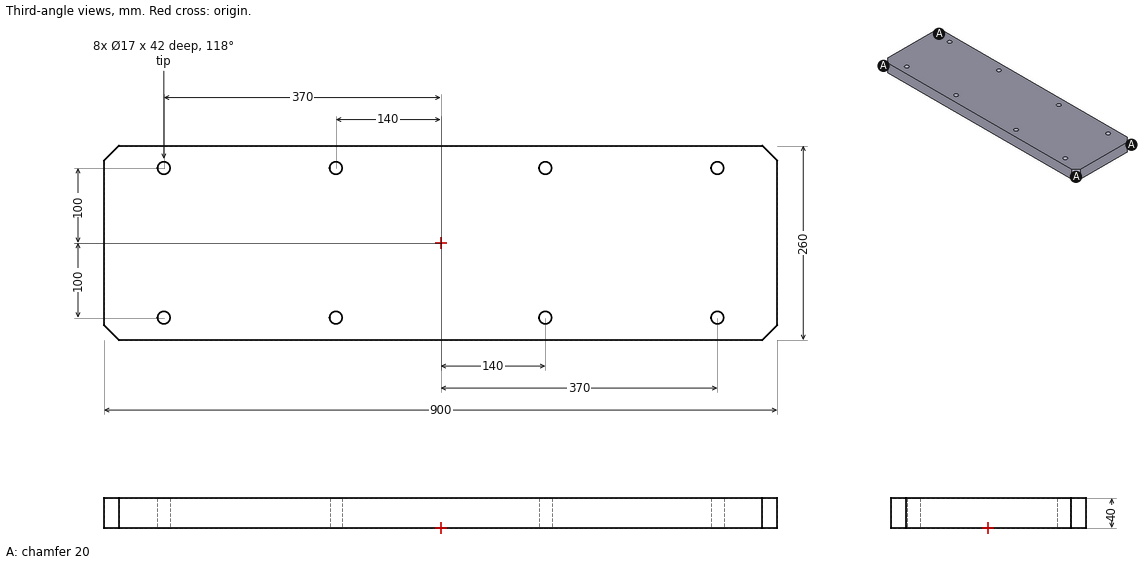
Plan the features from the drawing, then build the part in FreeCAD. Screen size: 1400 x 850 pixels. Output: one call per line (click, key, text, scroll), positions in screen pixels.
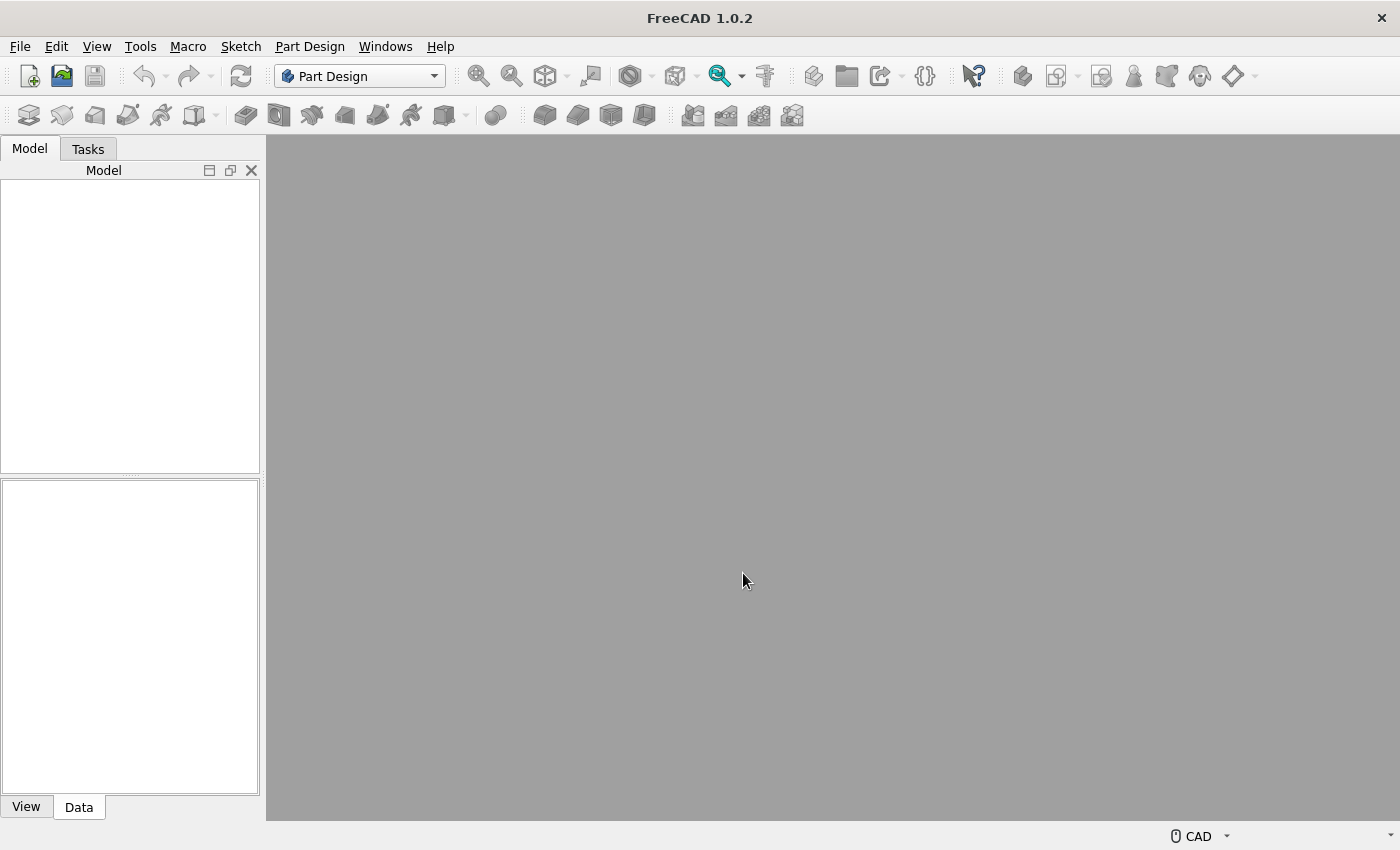
click(29, 76)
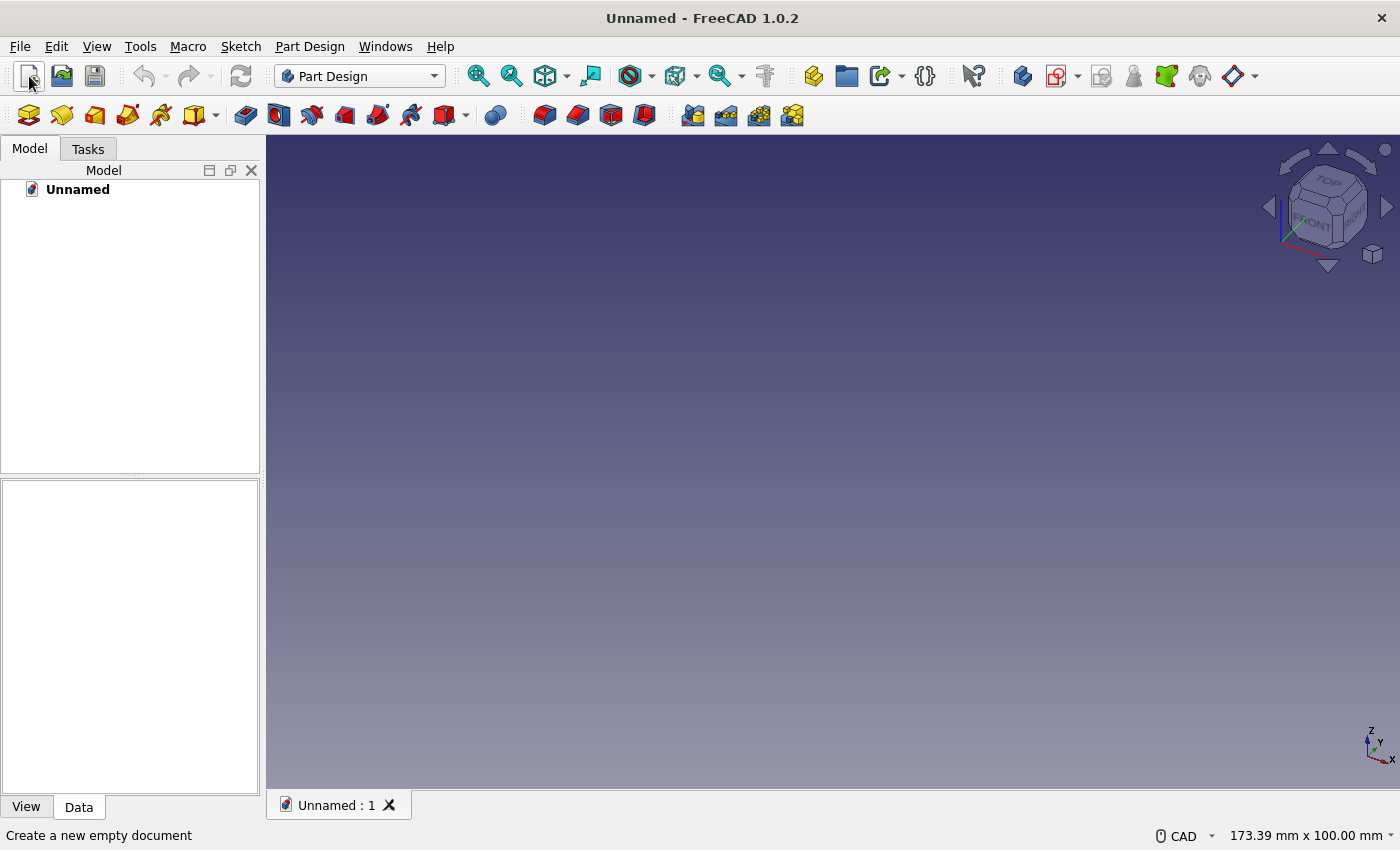
click(1056, 76)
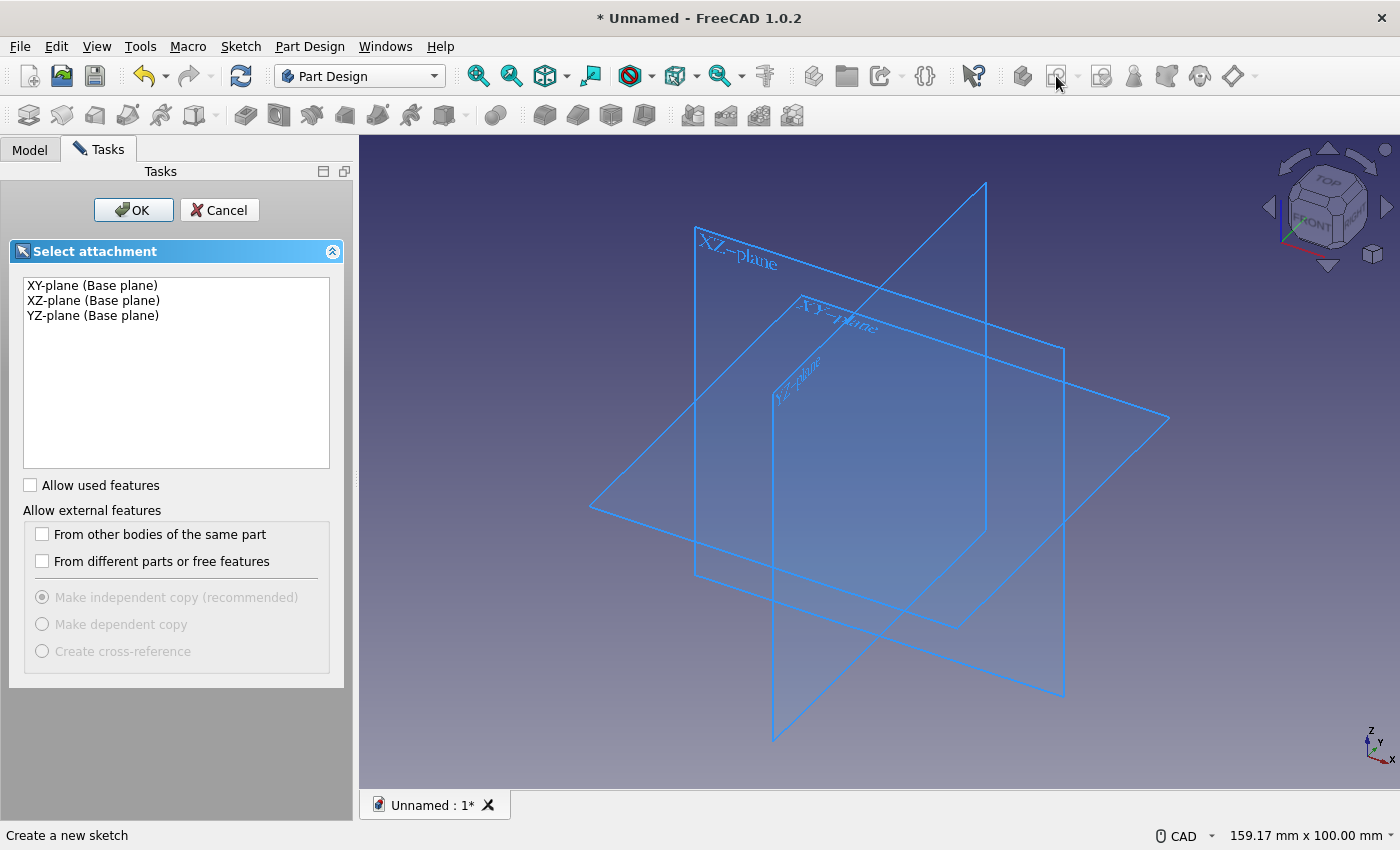
click(84, 286)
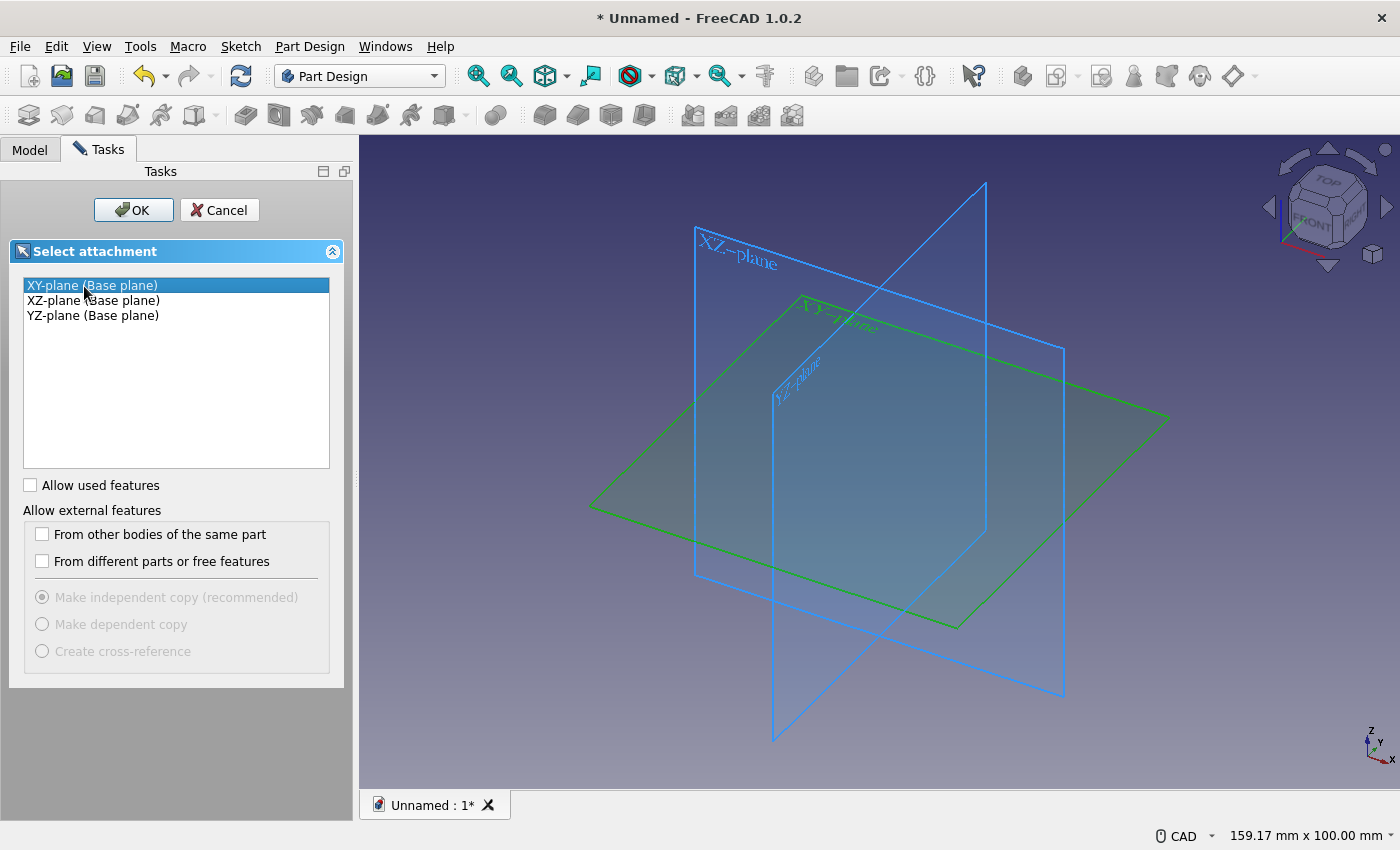
click(134, 210)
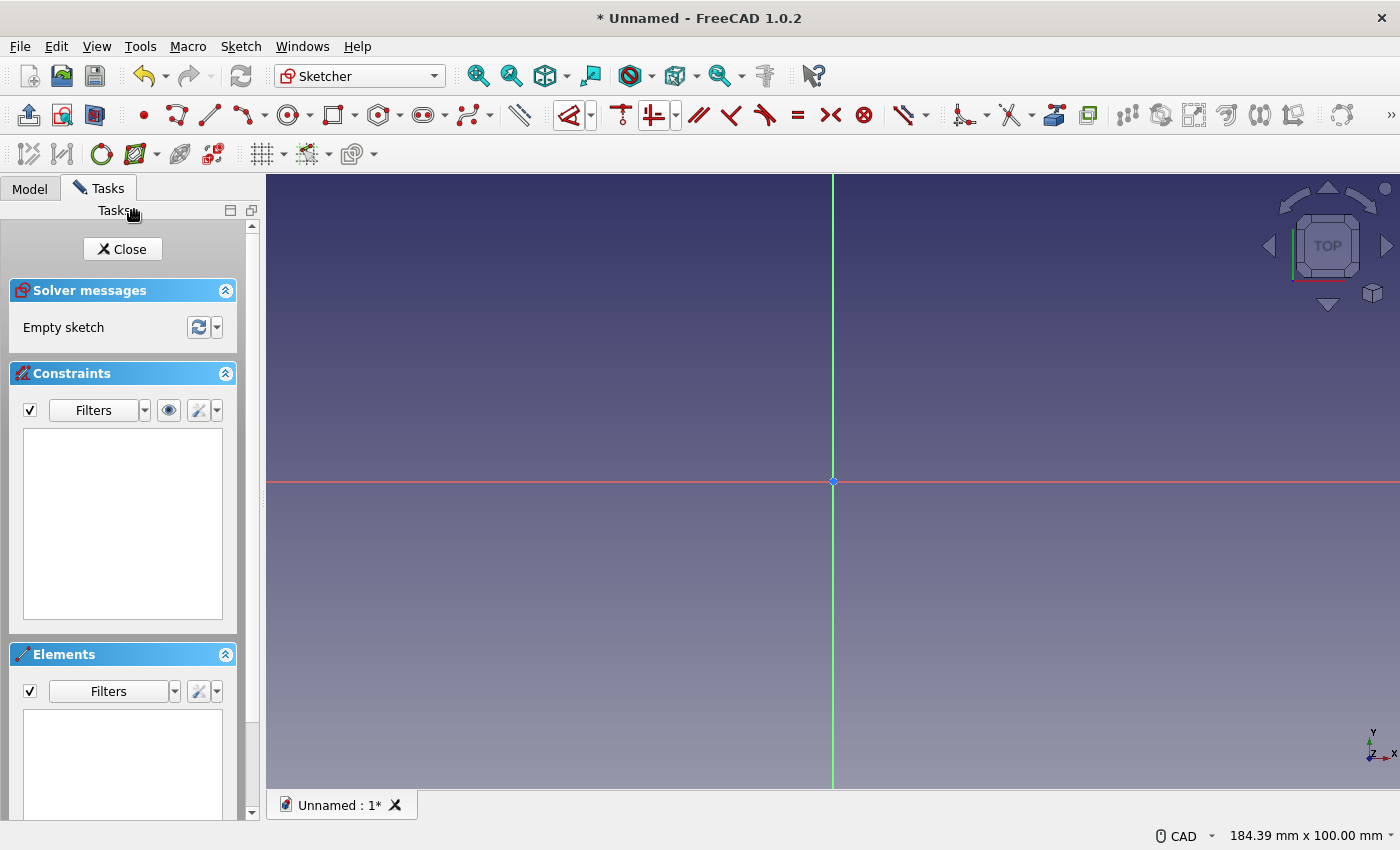
scroll(756, 482, down, 11)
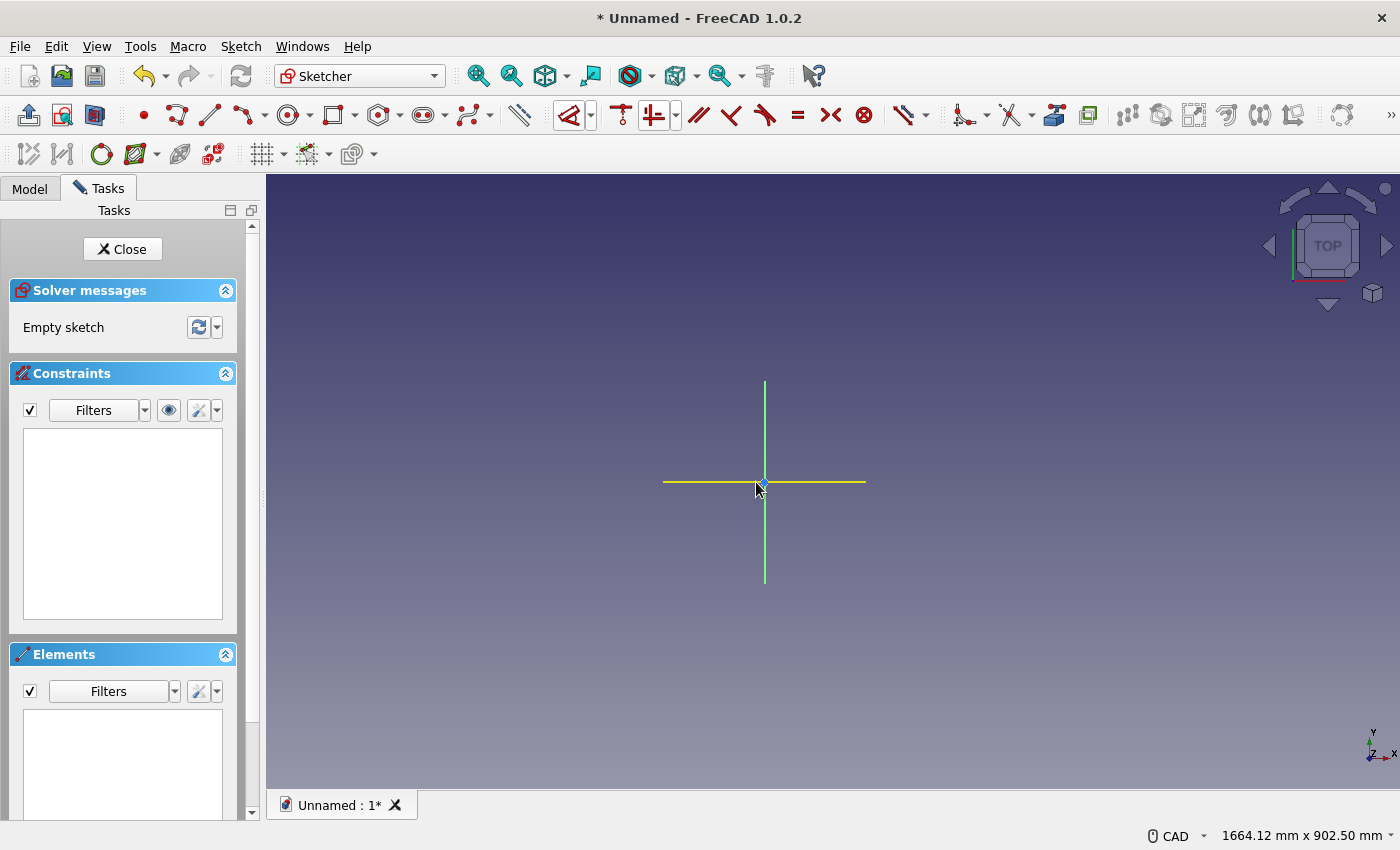
click(354, 116)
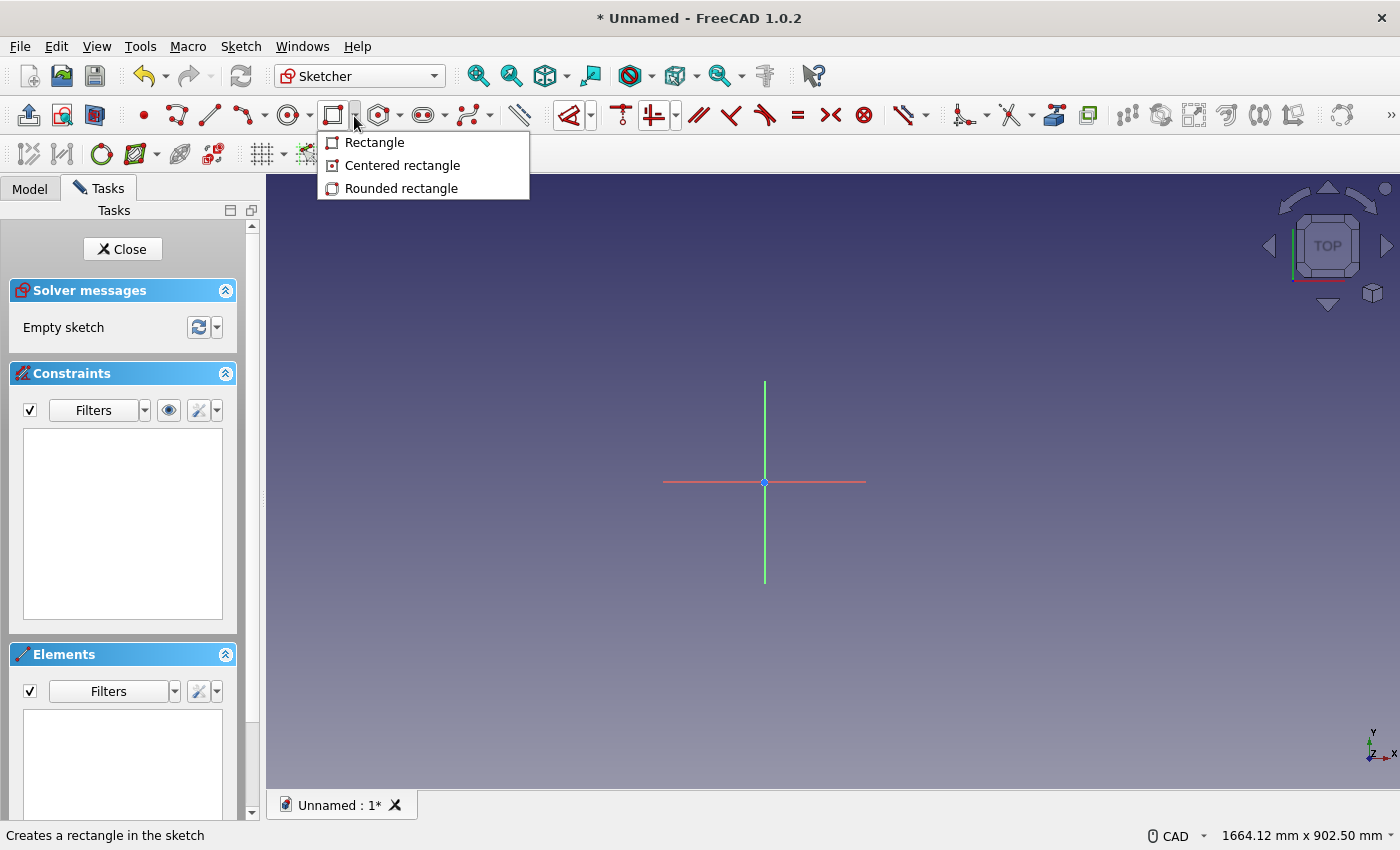
click(424, 166)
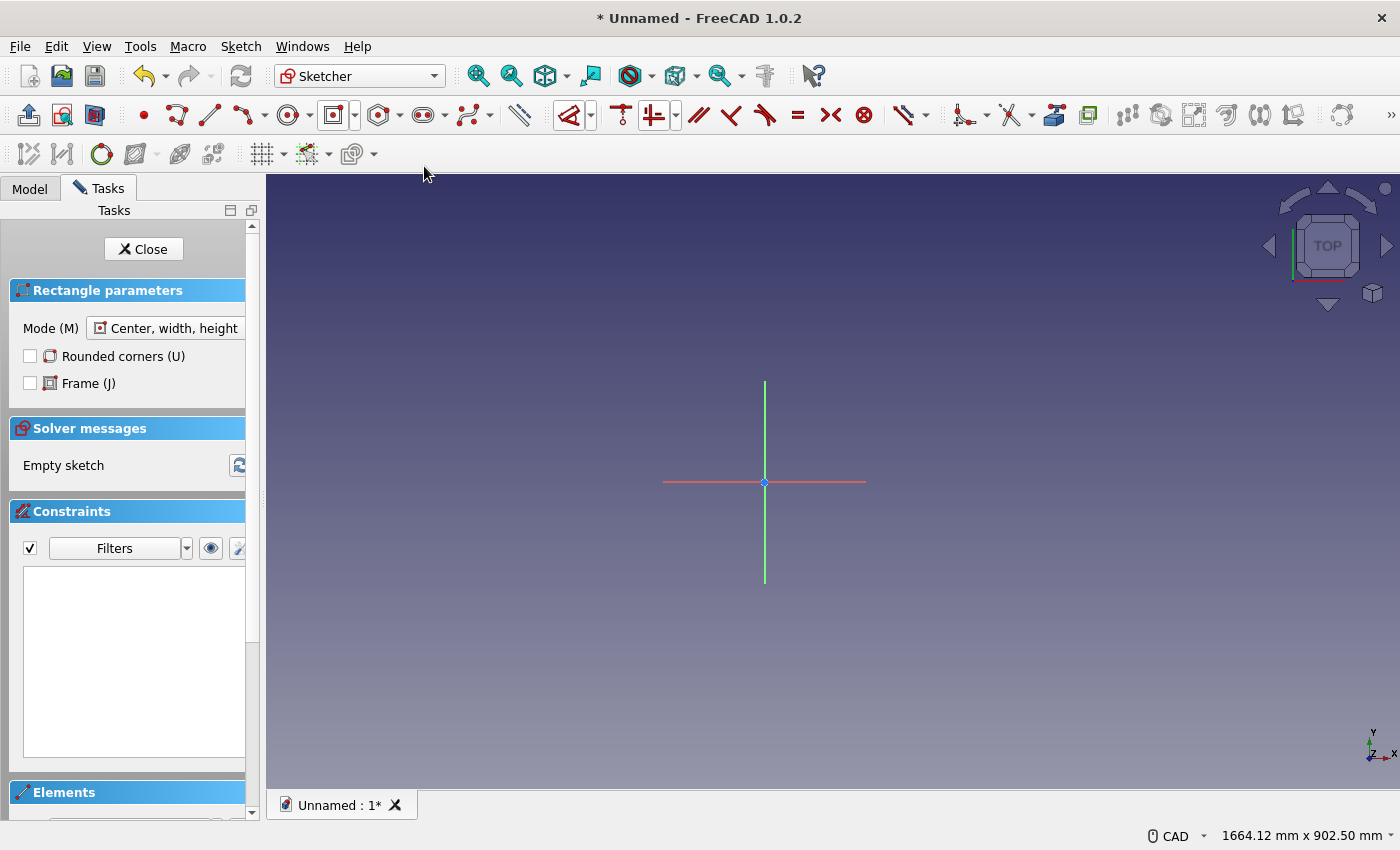
click(765, 482)
click(1072, 394)
key(Escape)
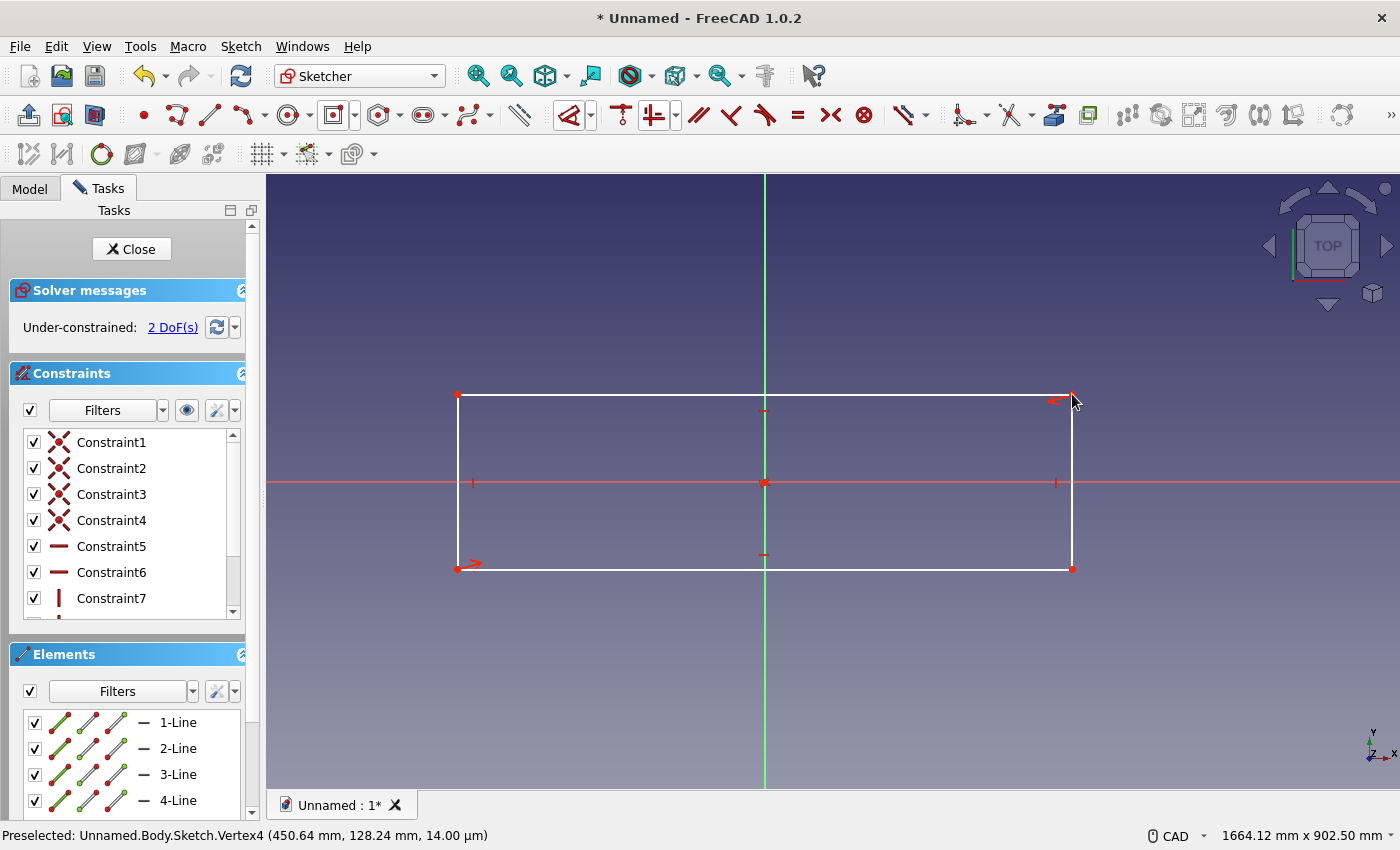
click(642, 570)